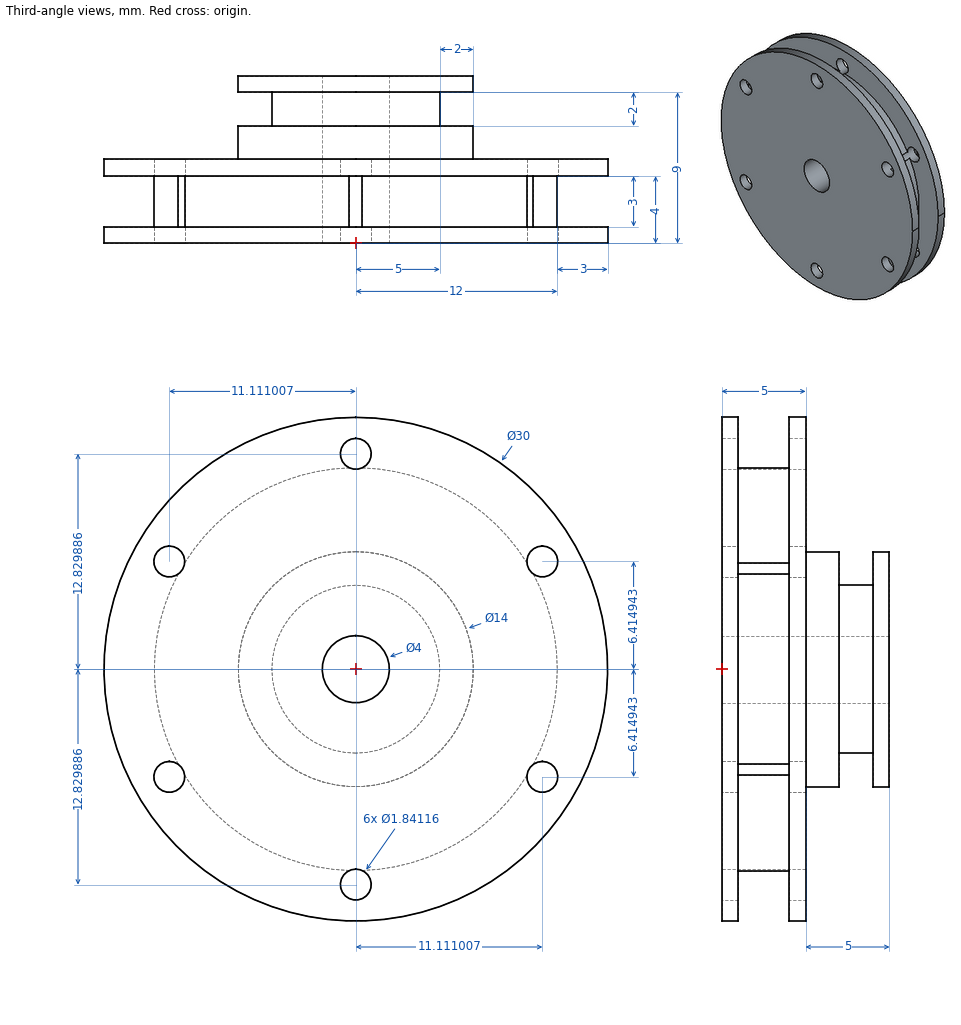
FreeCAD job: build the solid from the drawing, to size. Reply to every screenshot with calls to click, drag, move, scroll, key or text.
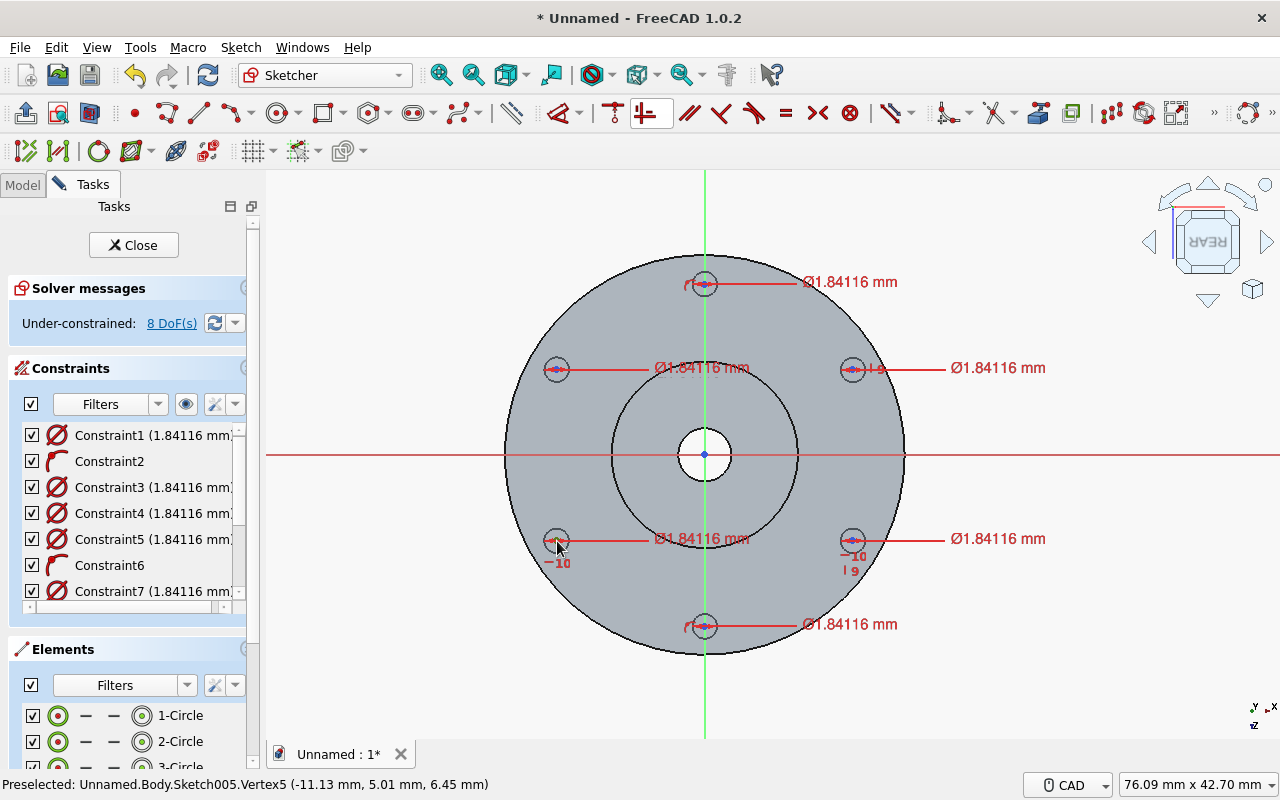
click(557, 370)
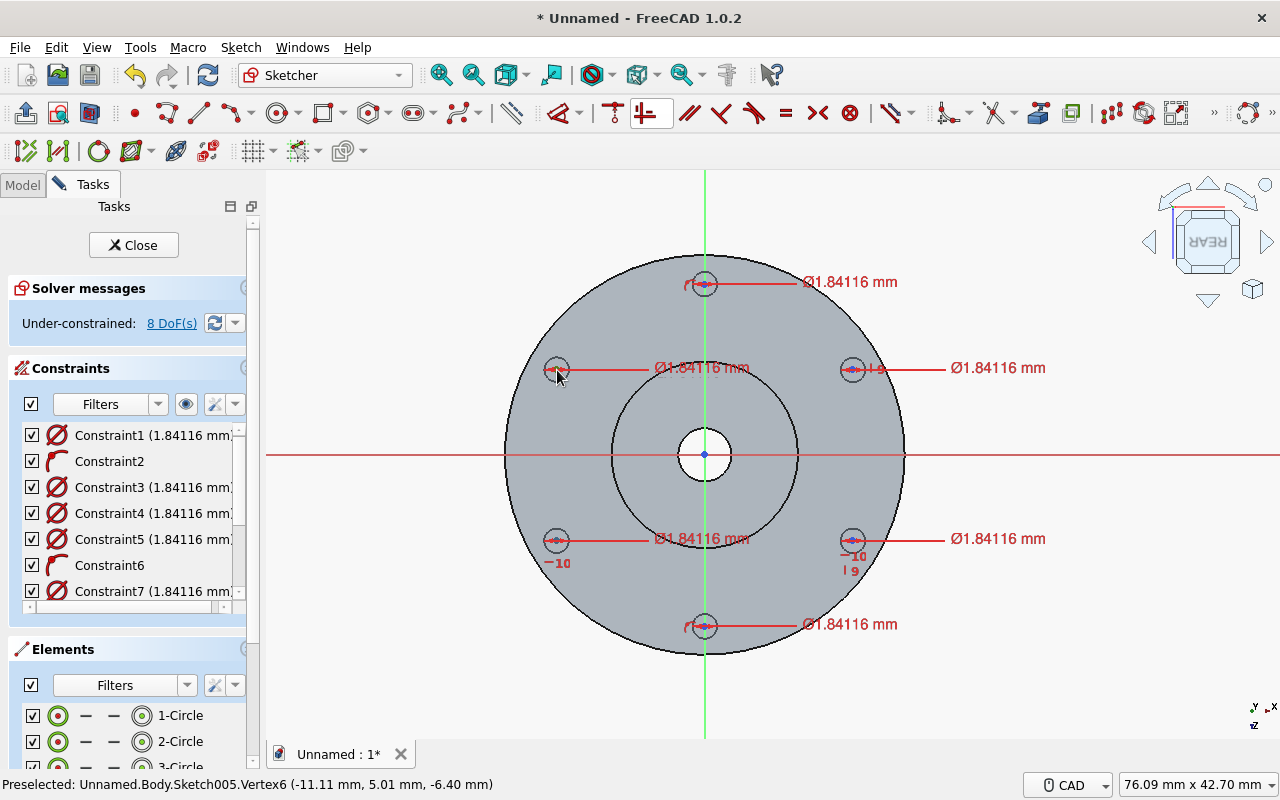
click(668, 114)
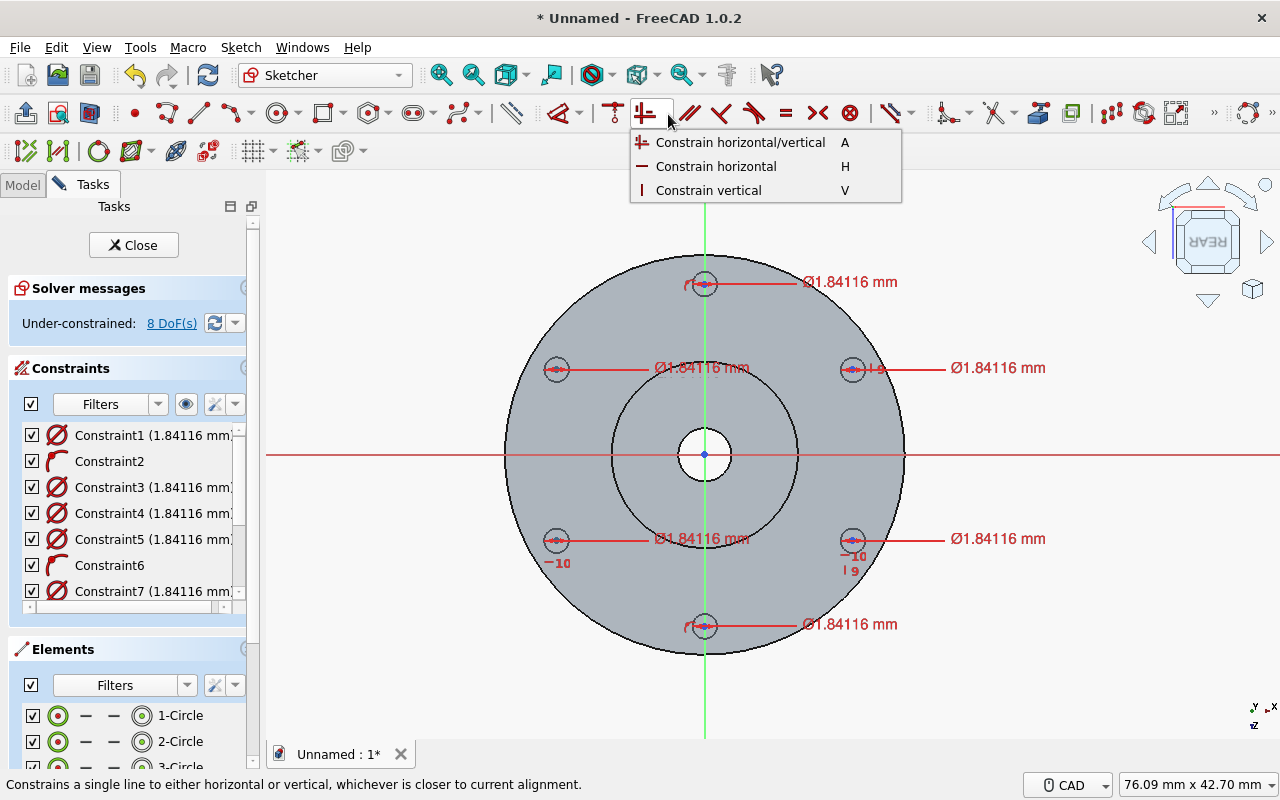
click(766, 190)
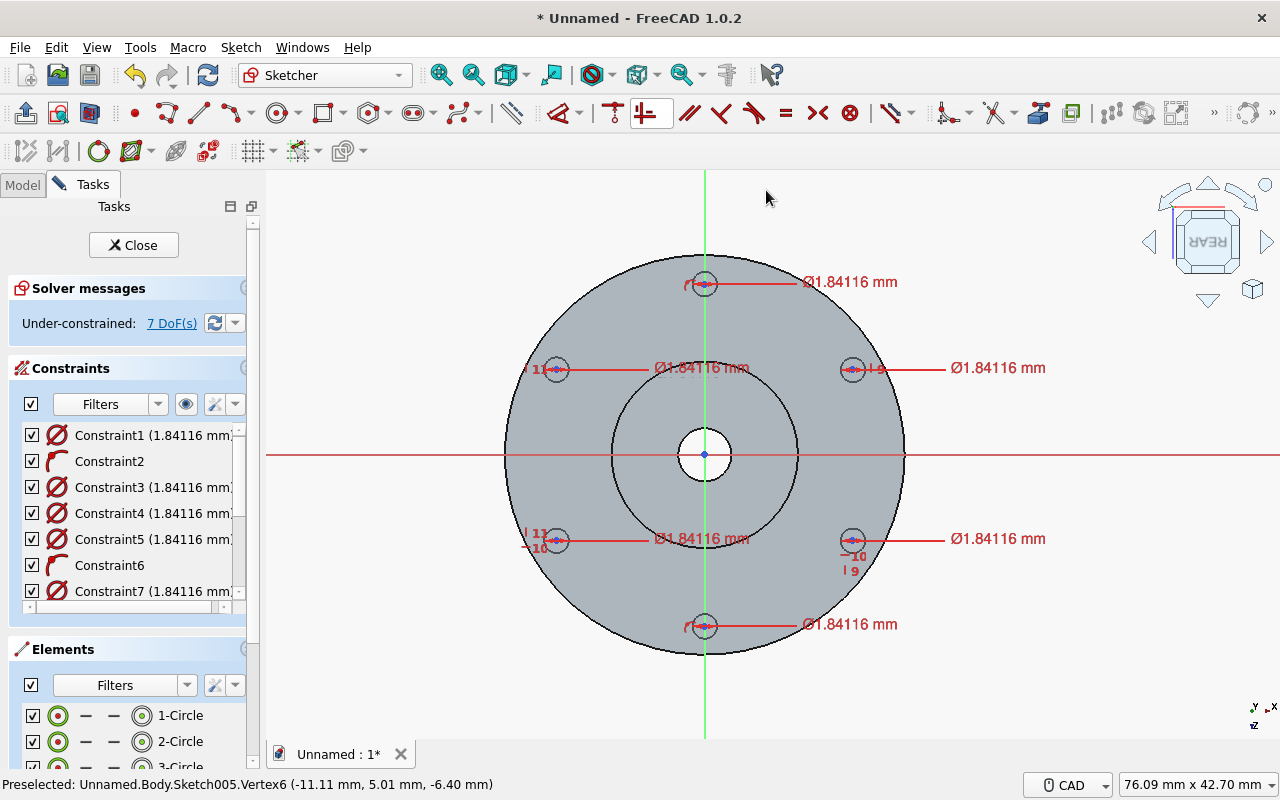
click(853, 370)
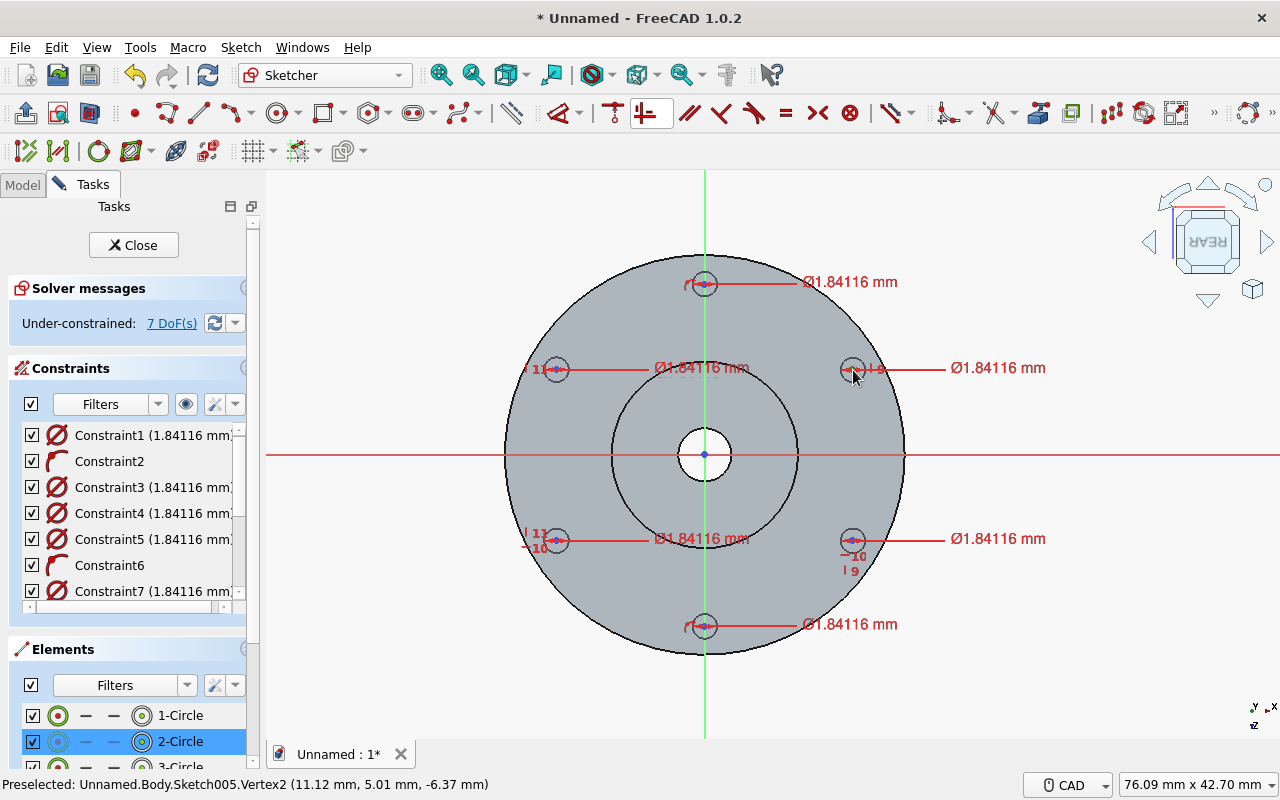
click(557, 370)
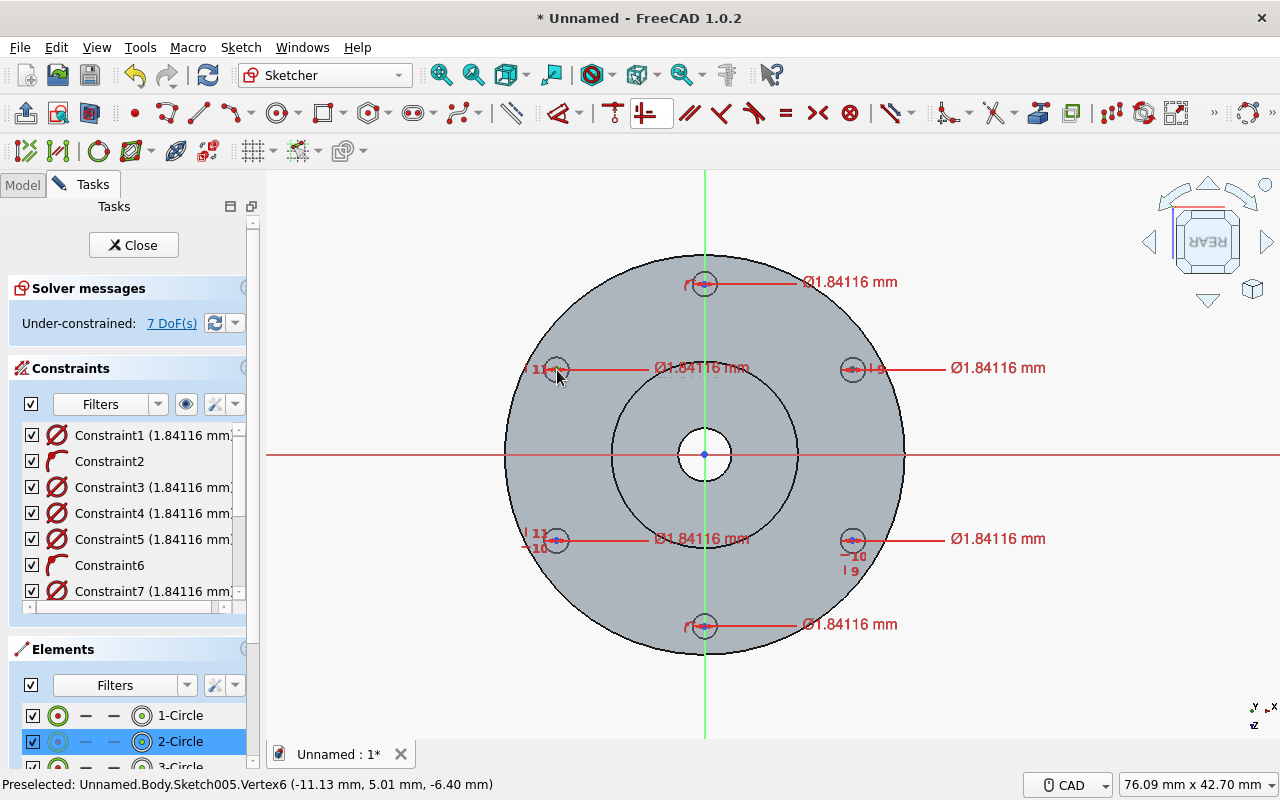
key(h)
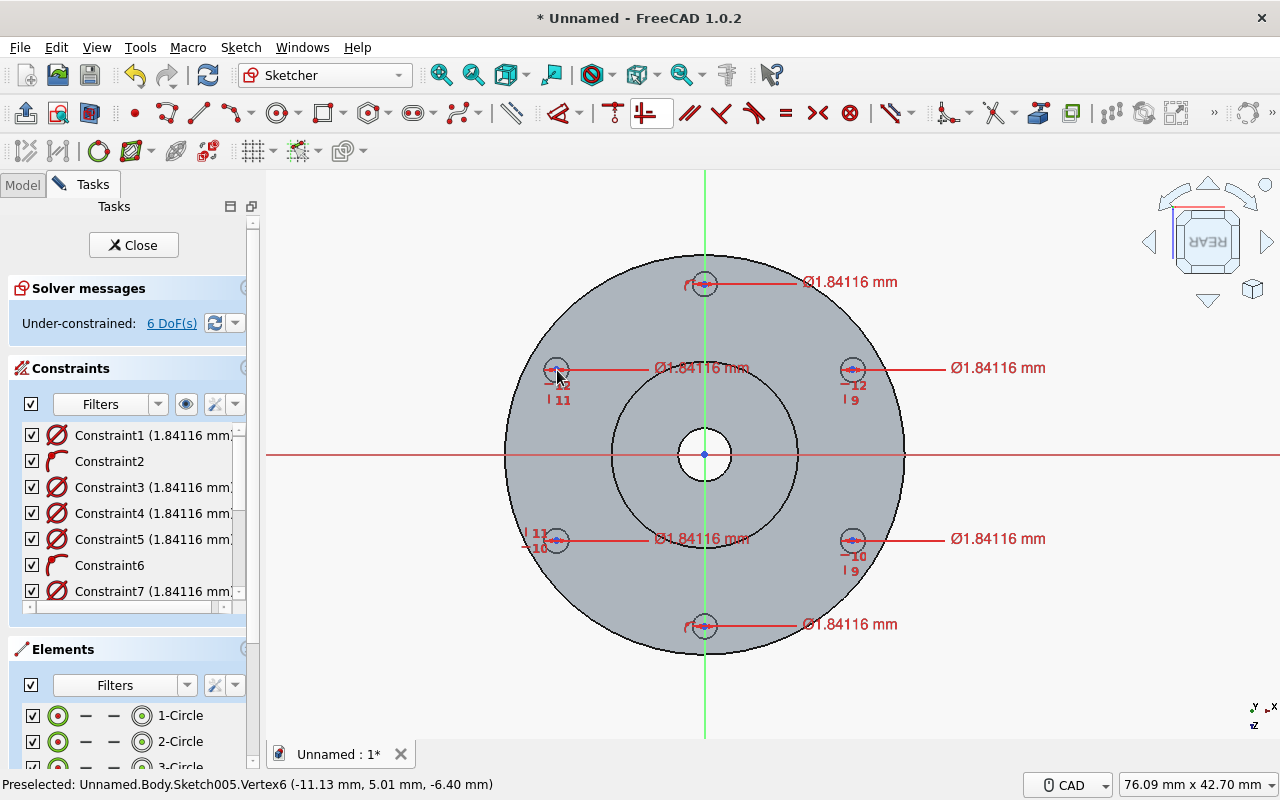
click(558, 114)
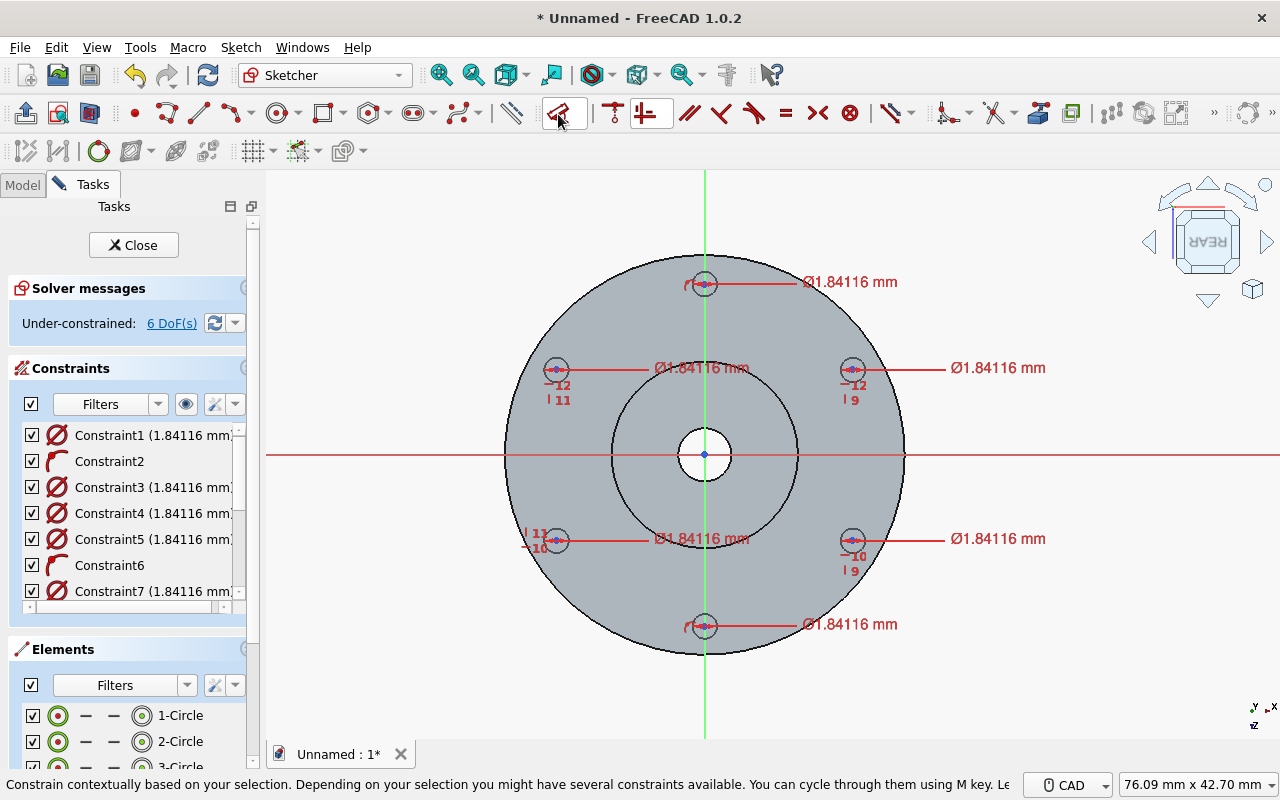
click(853, 370)
click(887, 412)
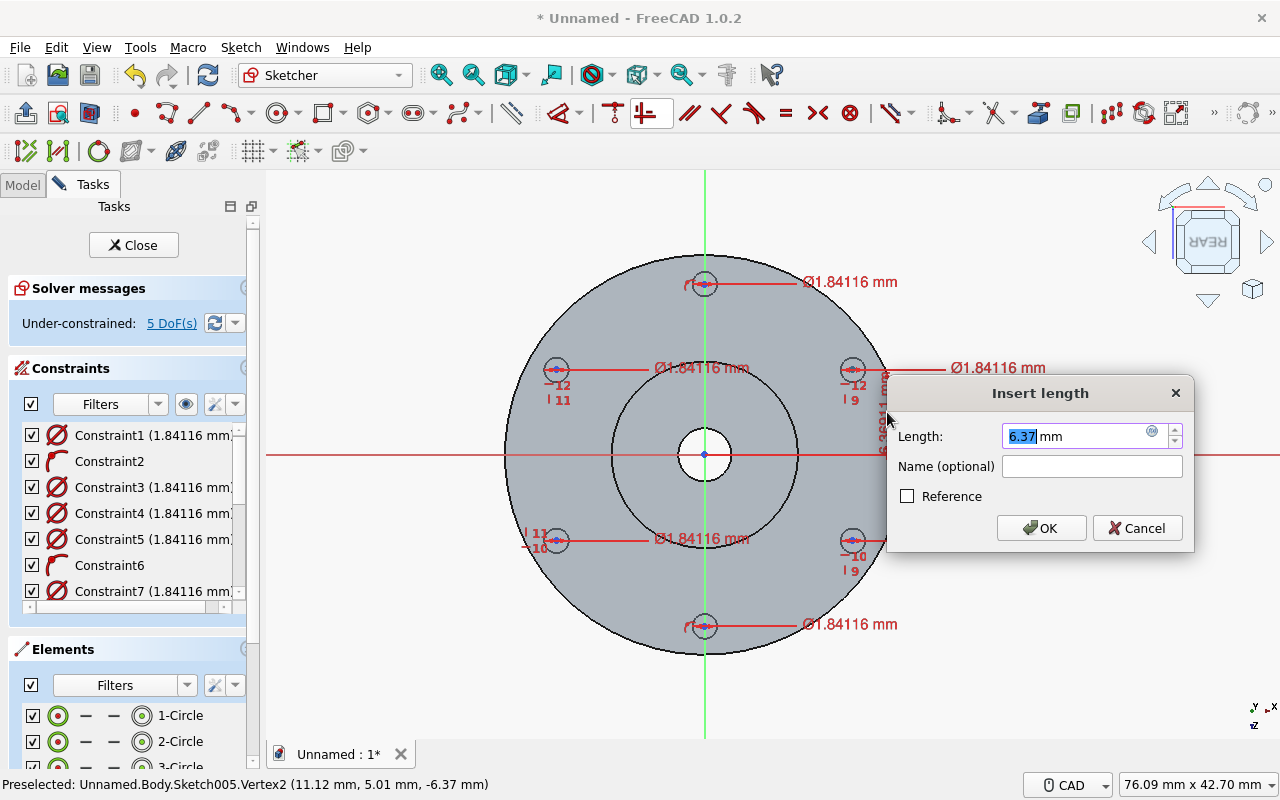
text(6.414943)
key(Return)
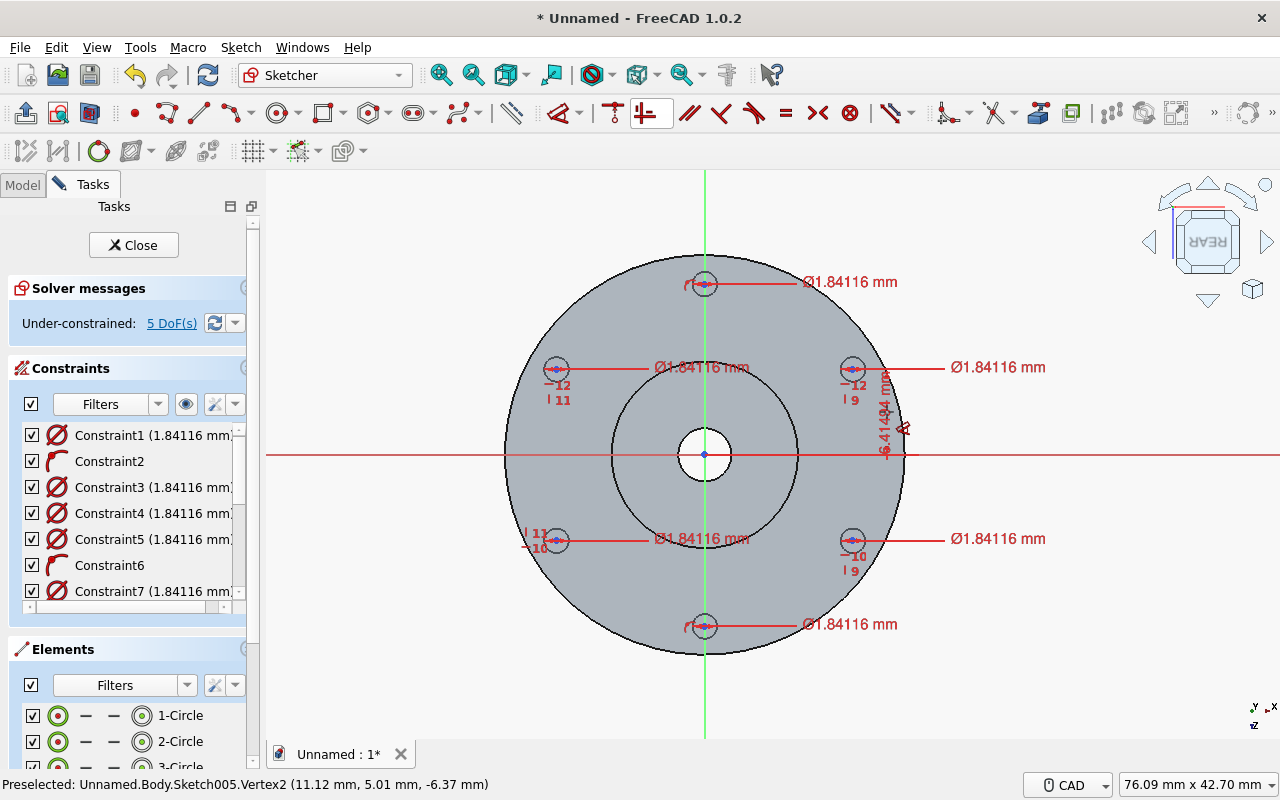
click(853, 541)
click(887, 498)